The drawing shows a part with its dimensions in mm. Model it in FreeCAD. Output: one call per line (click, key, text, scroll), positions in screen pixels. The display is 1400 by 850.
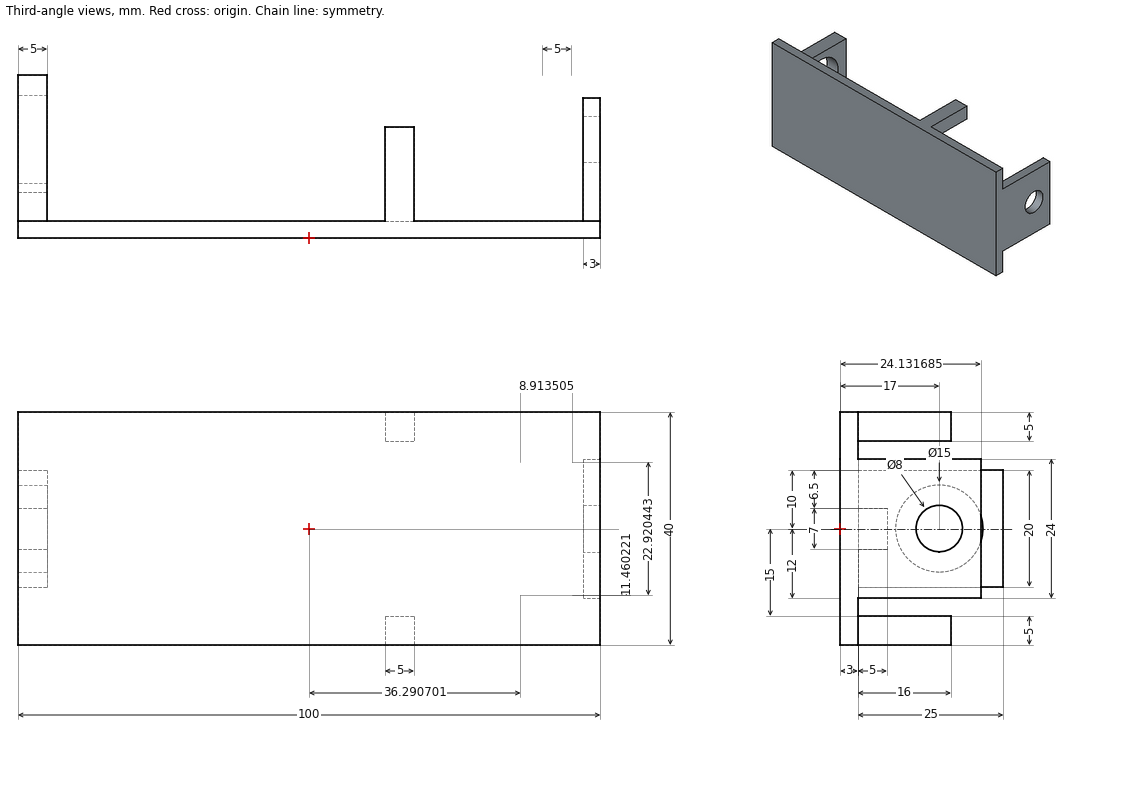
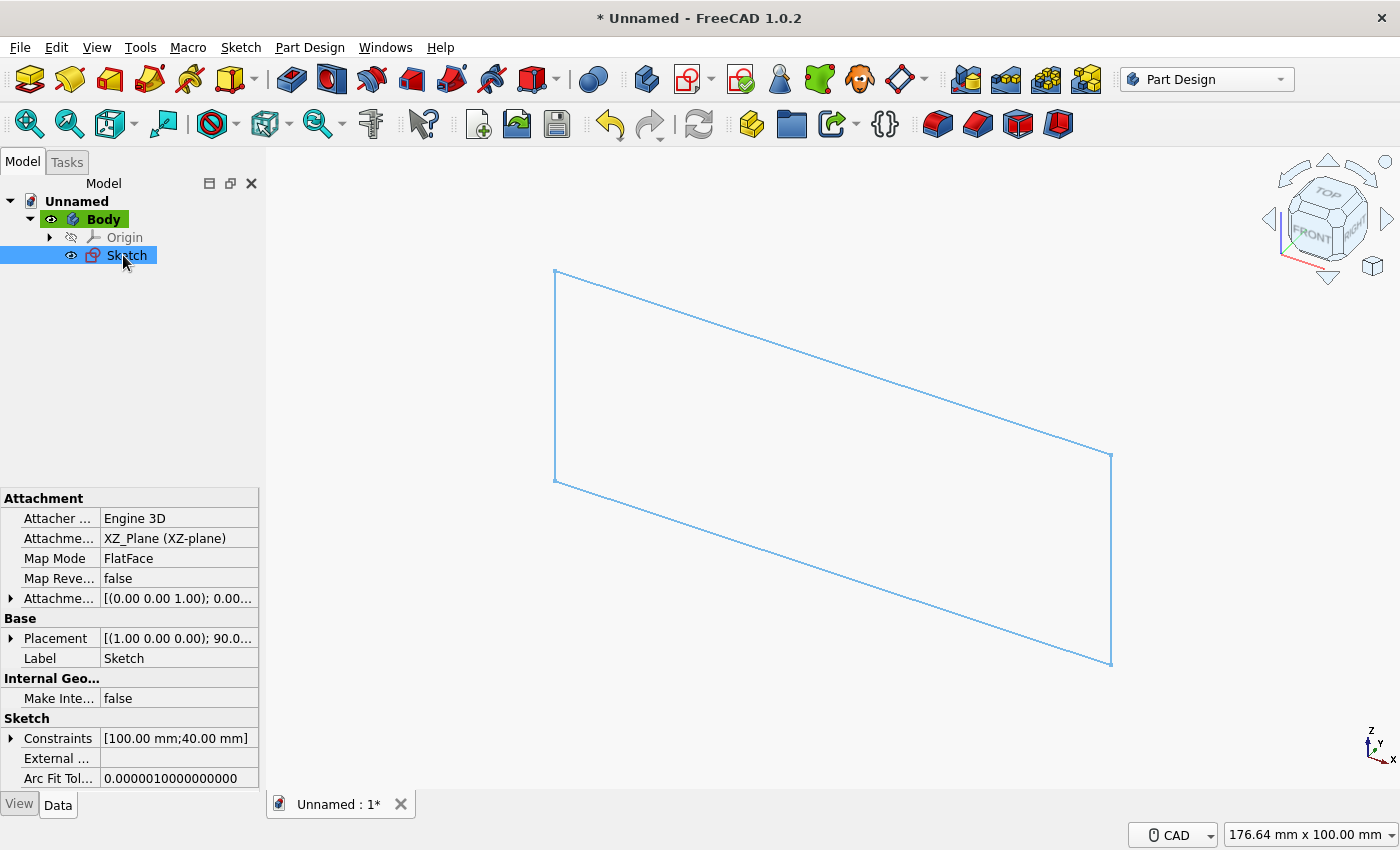
click(30, 80)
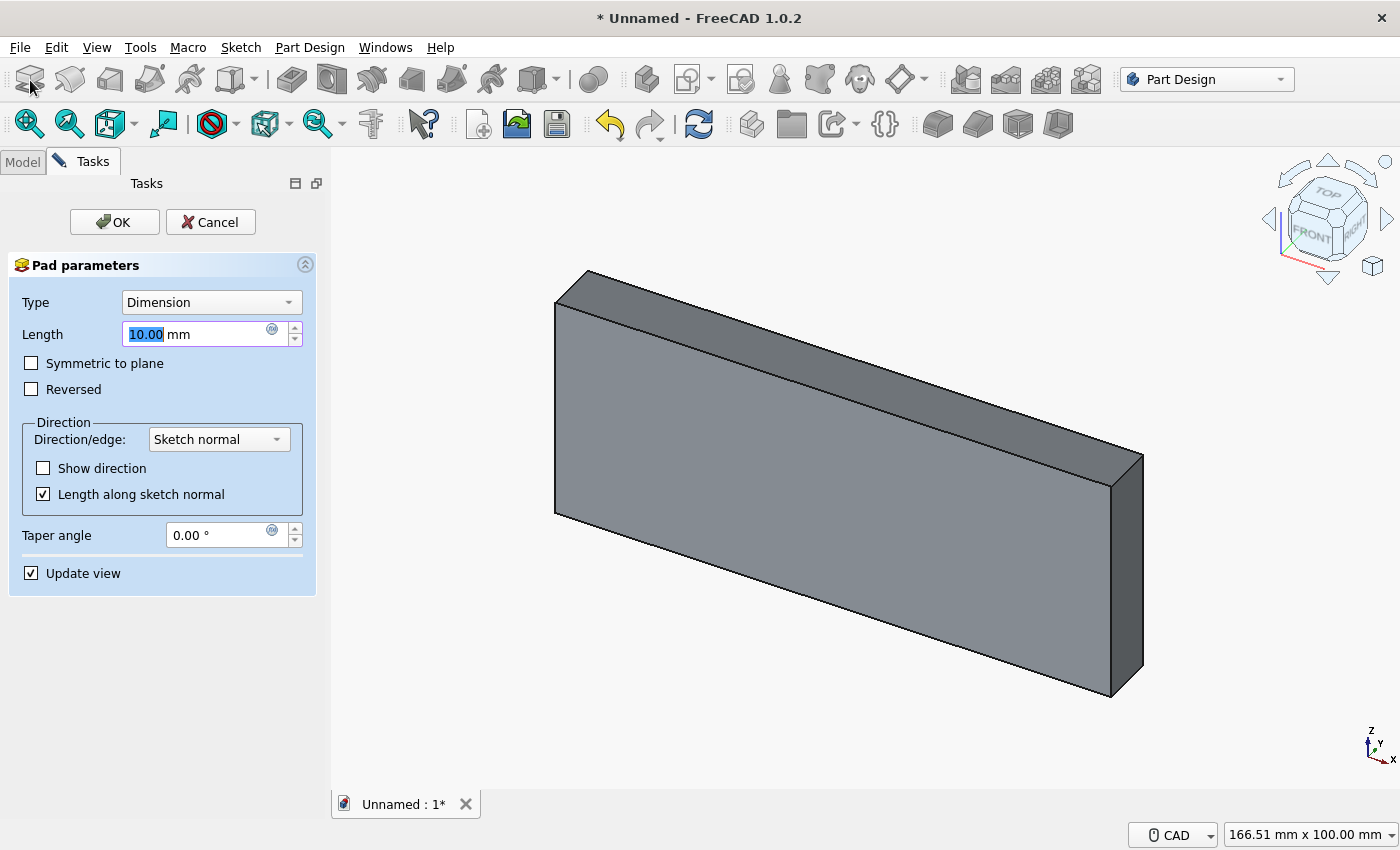
text(3)
key(Tab)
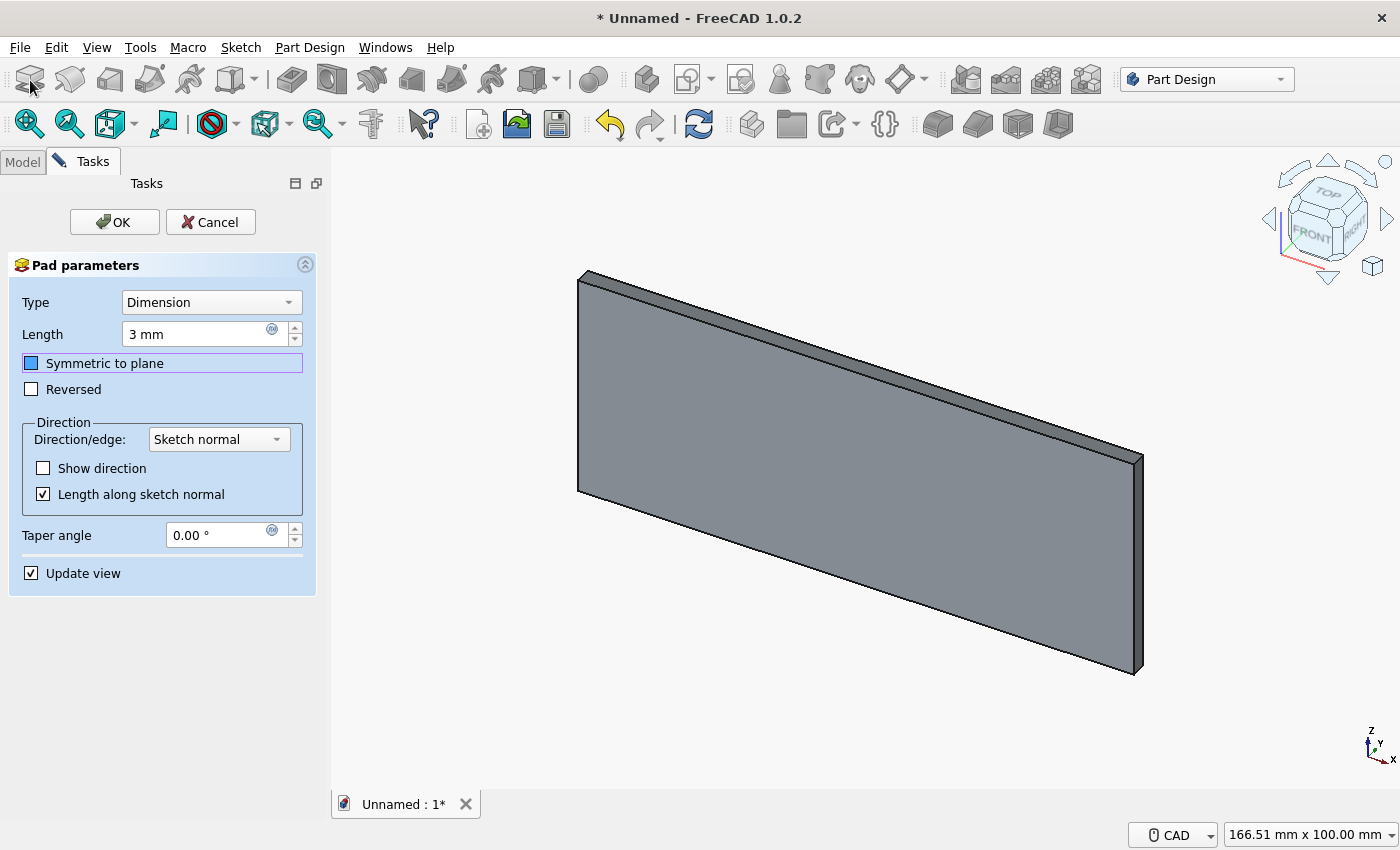
click(30, 389)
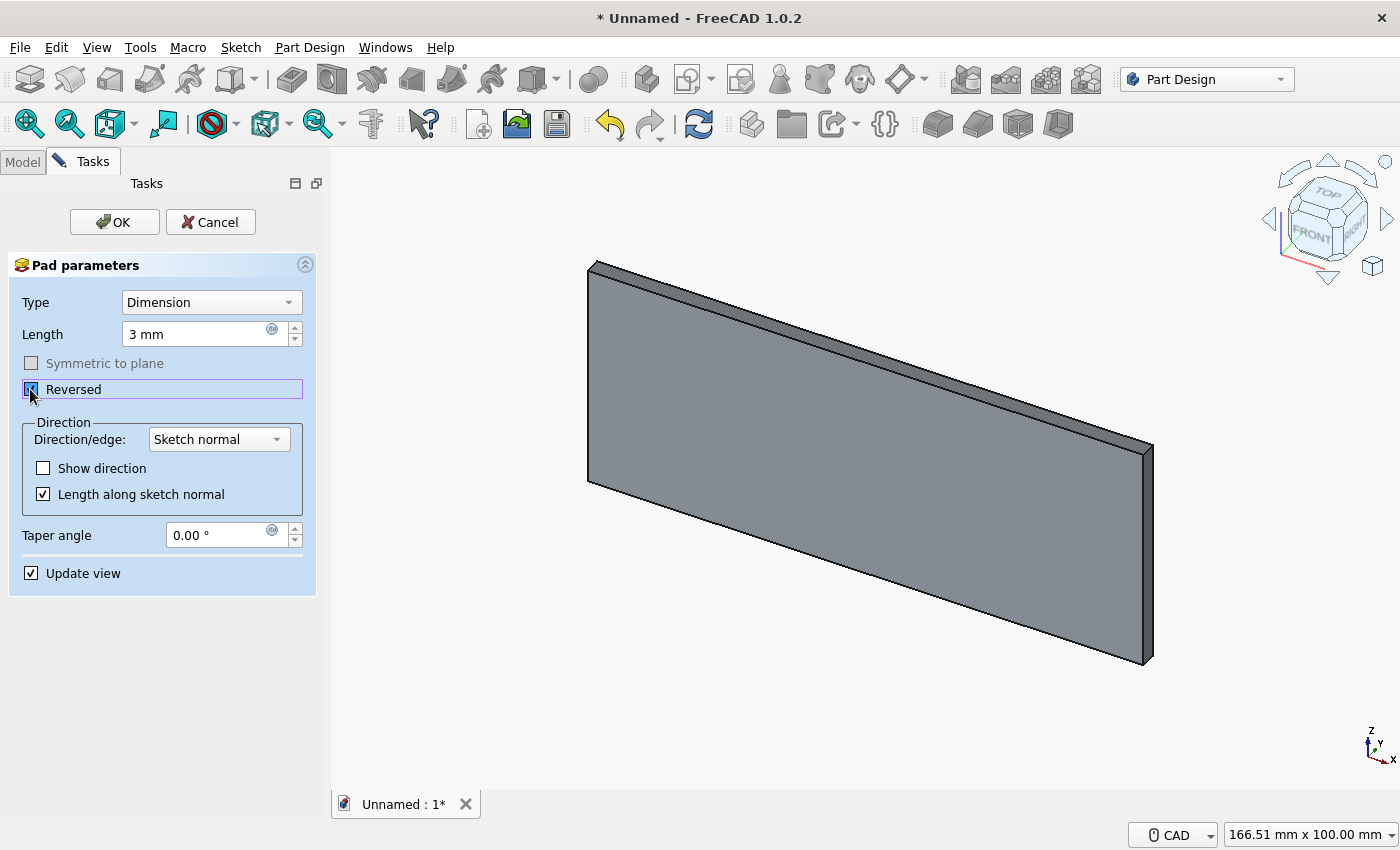
click(115, 222)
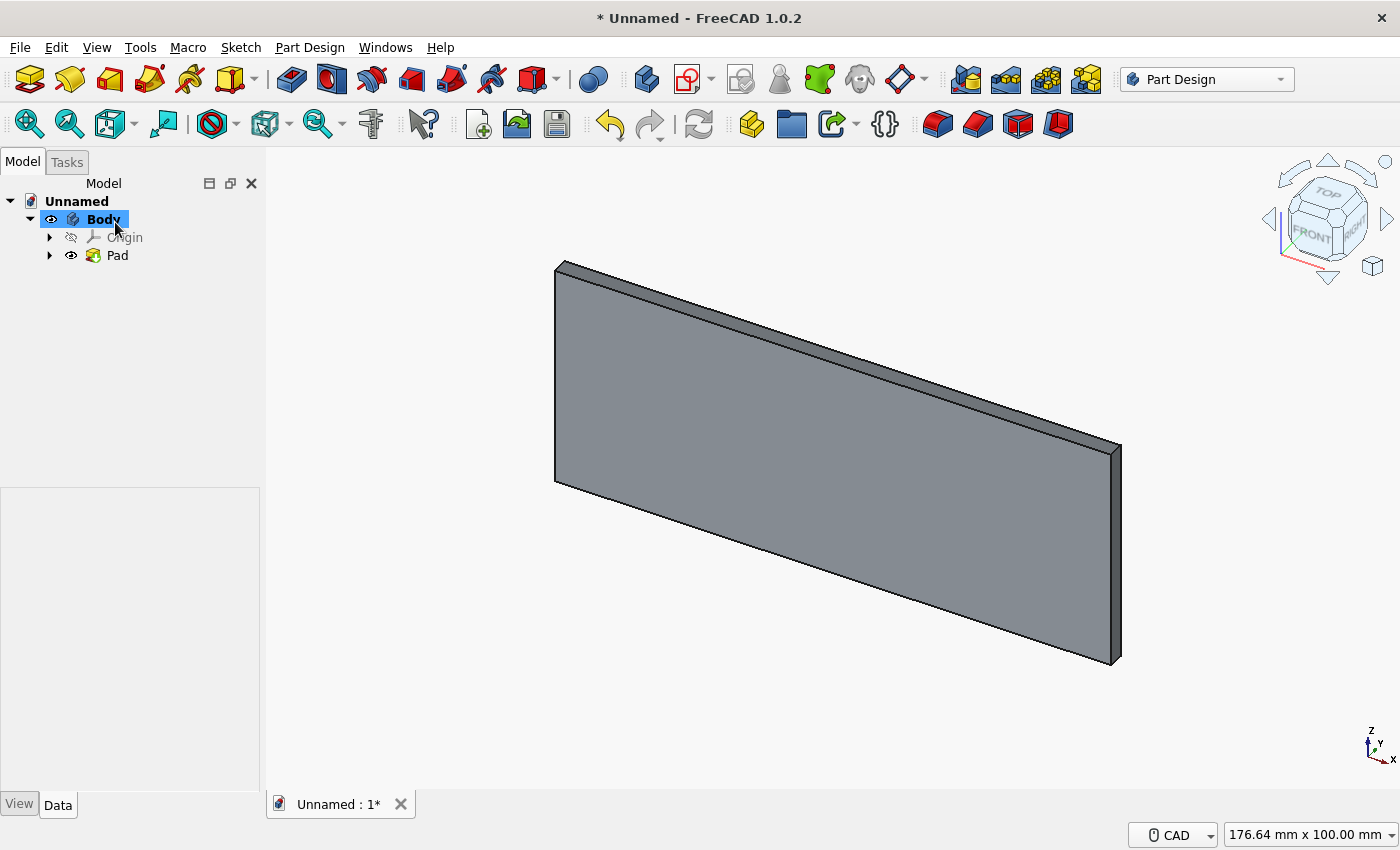
click(50, 237)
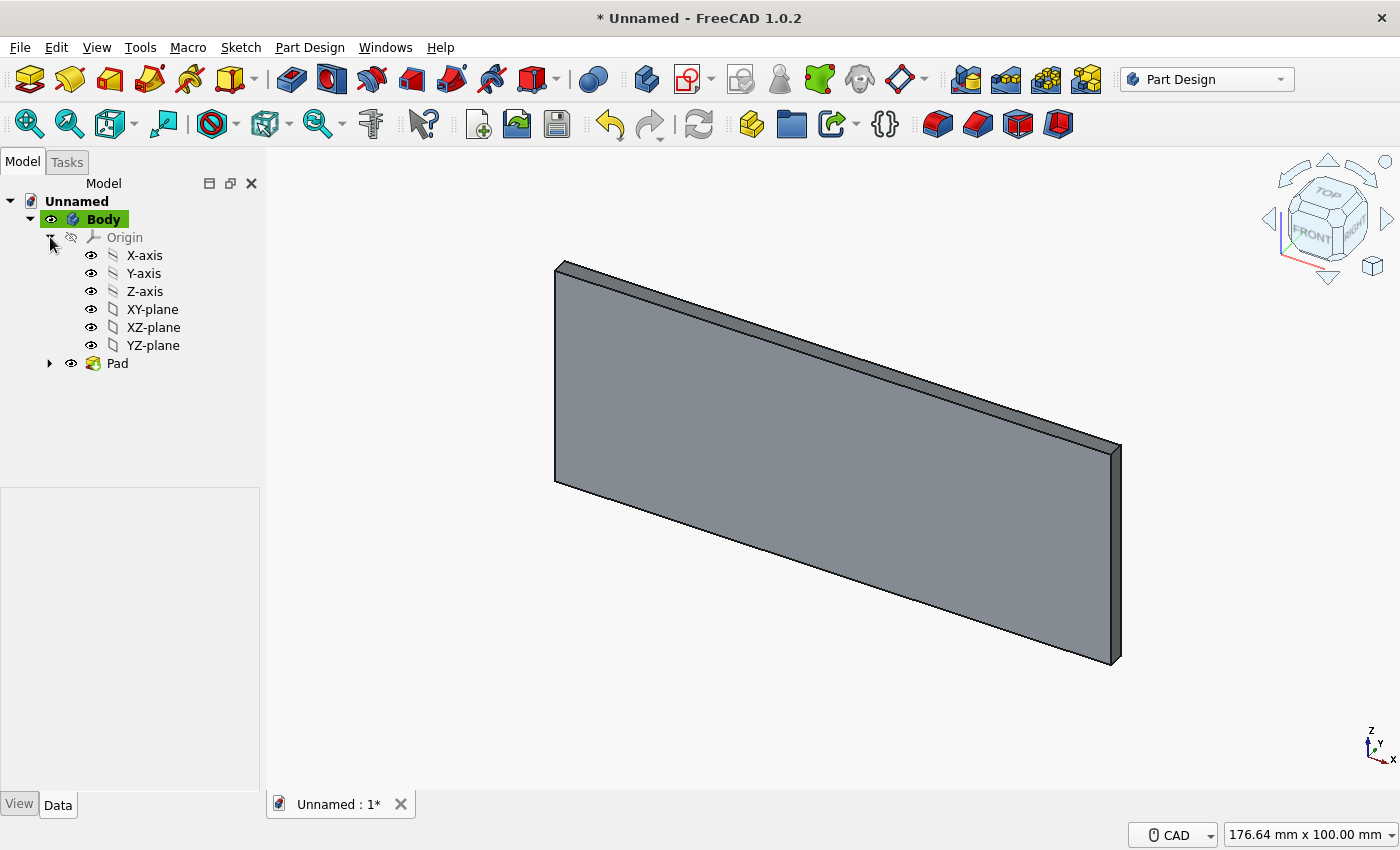
click(136, 345)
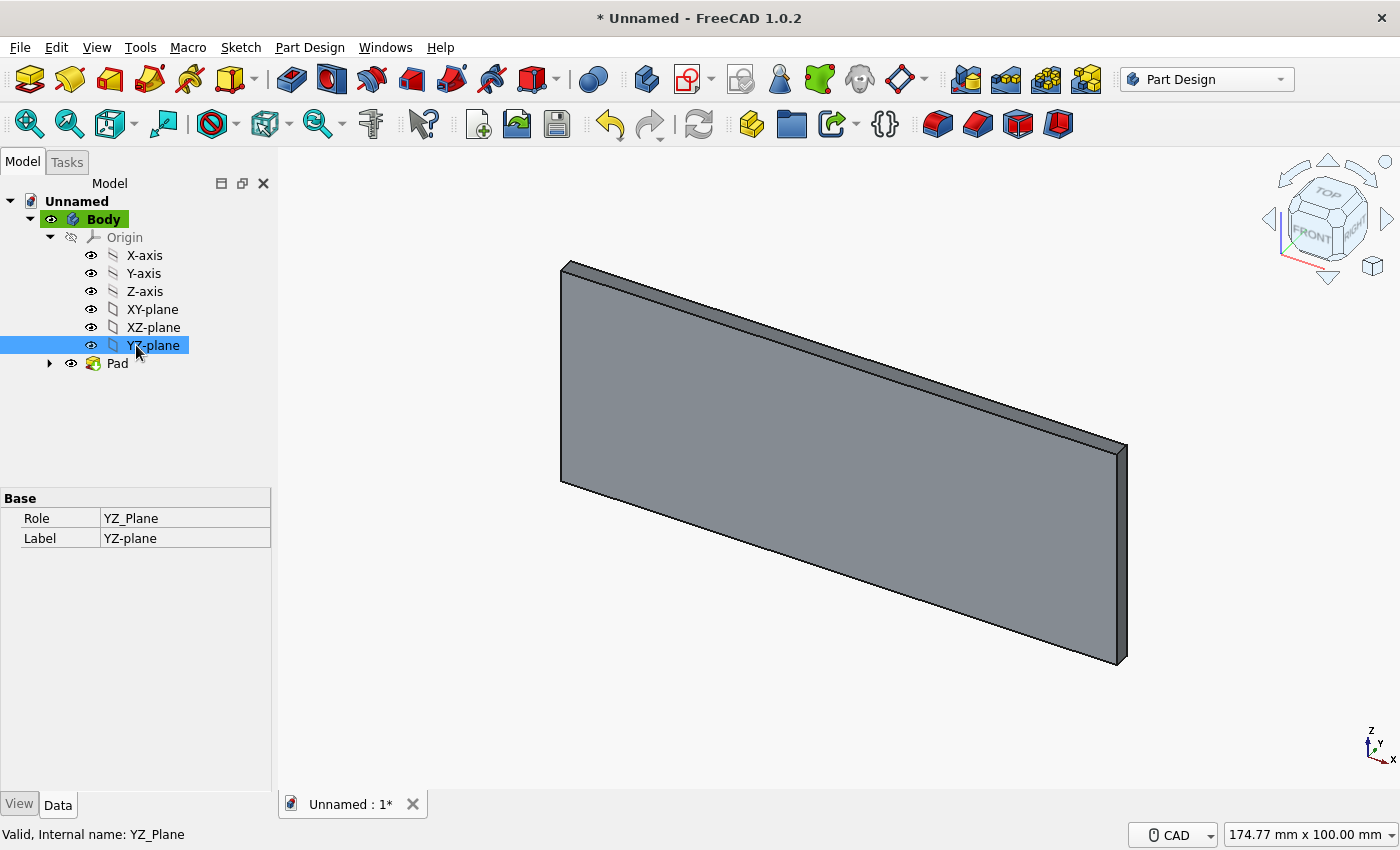
click(900, 80)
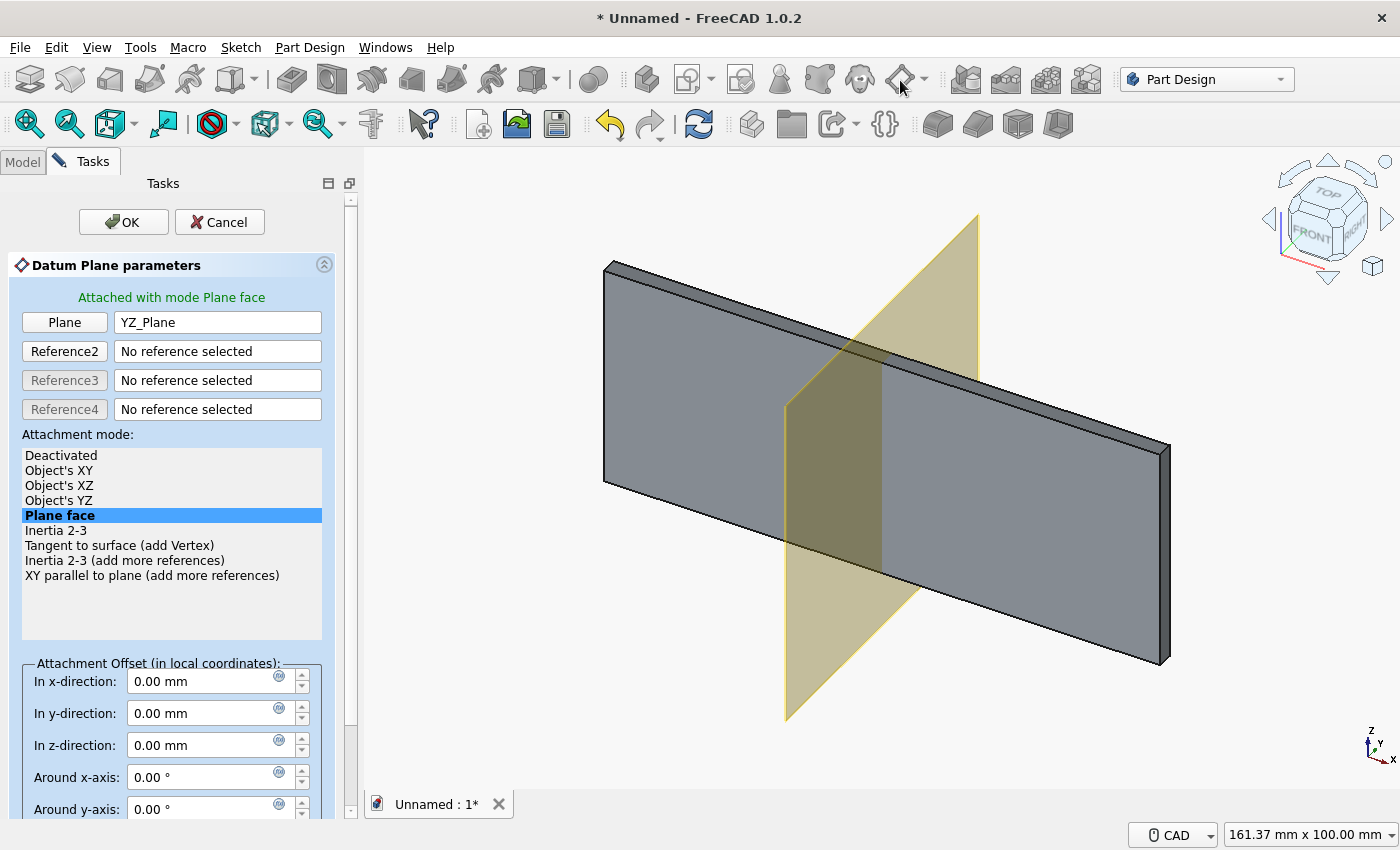
triple_click(210, 745)